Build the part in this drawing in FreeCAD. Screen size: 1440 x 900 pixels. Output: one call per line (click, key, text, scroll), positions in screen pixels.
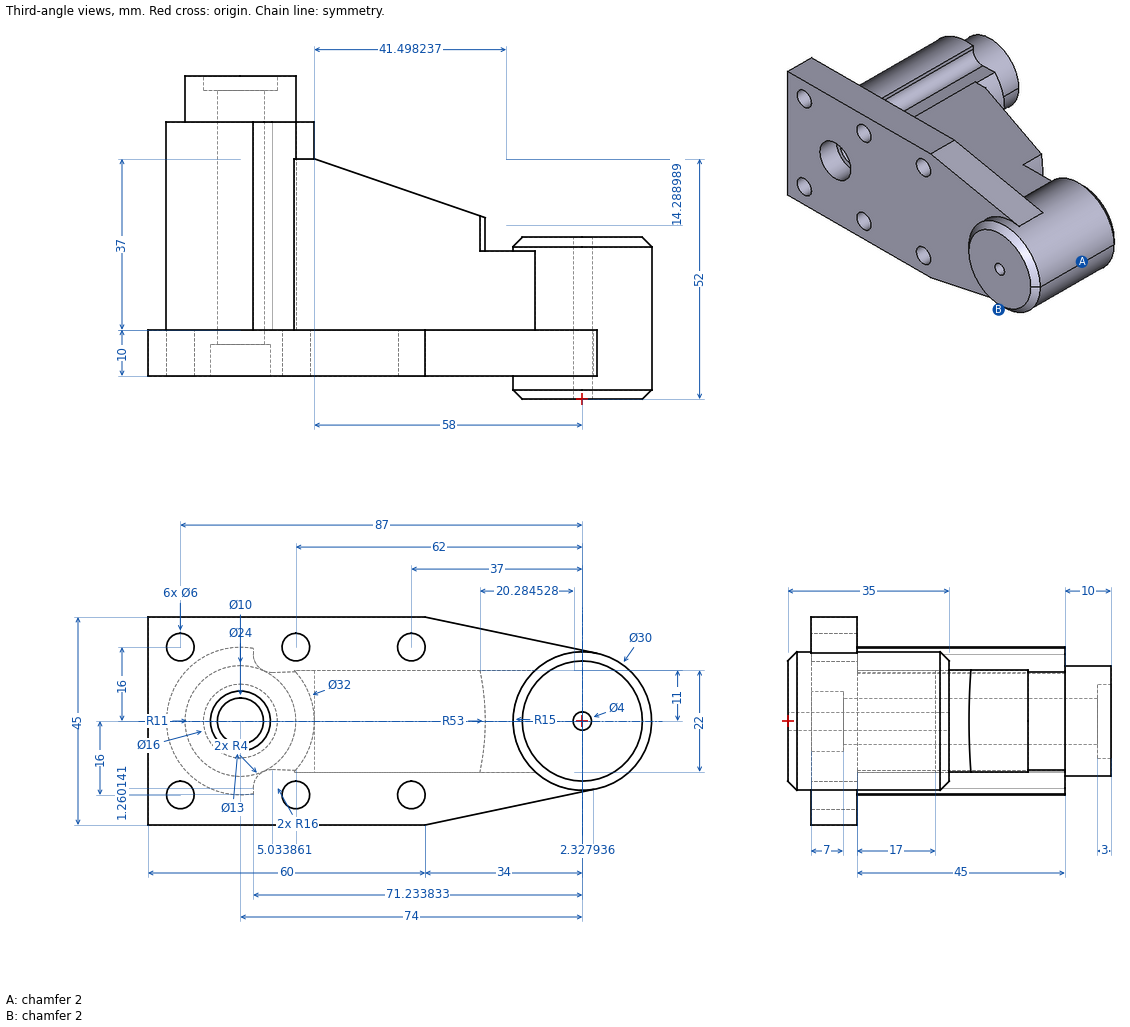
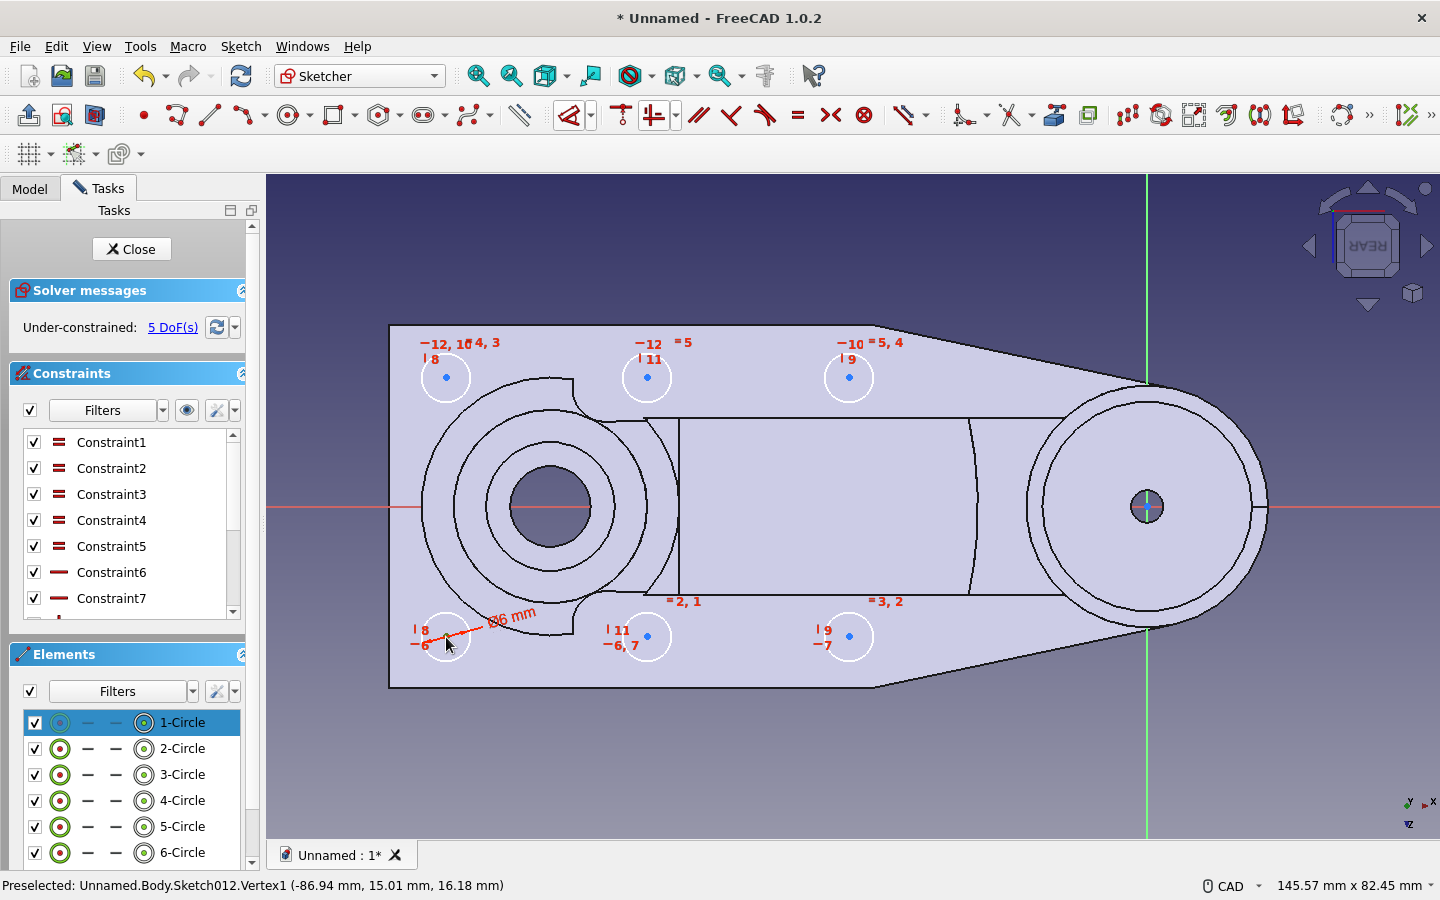
key(l)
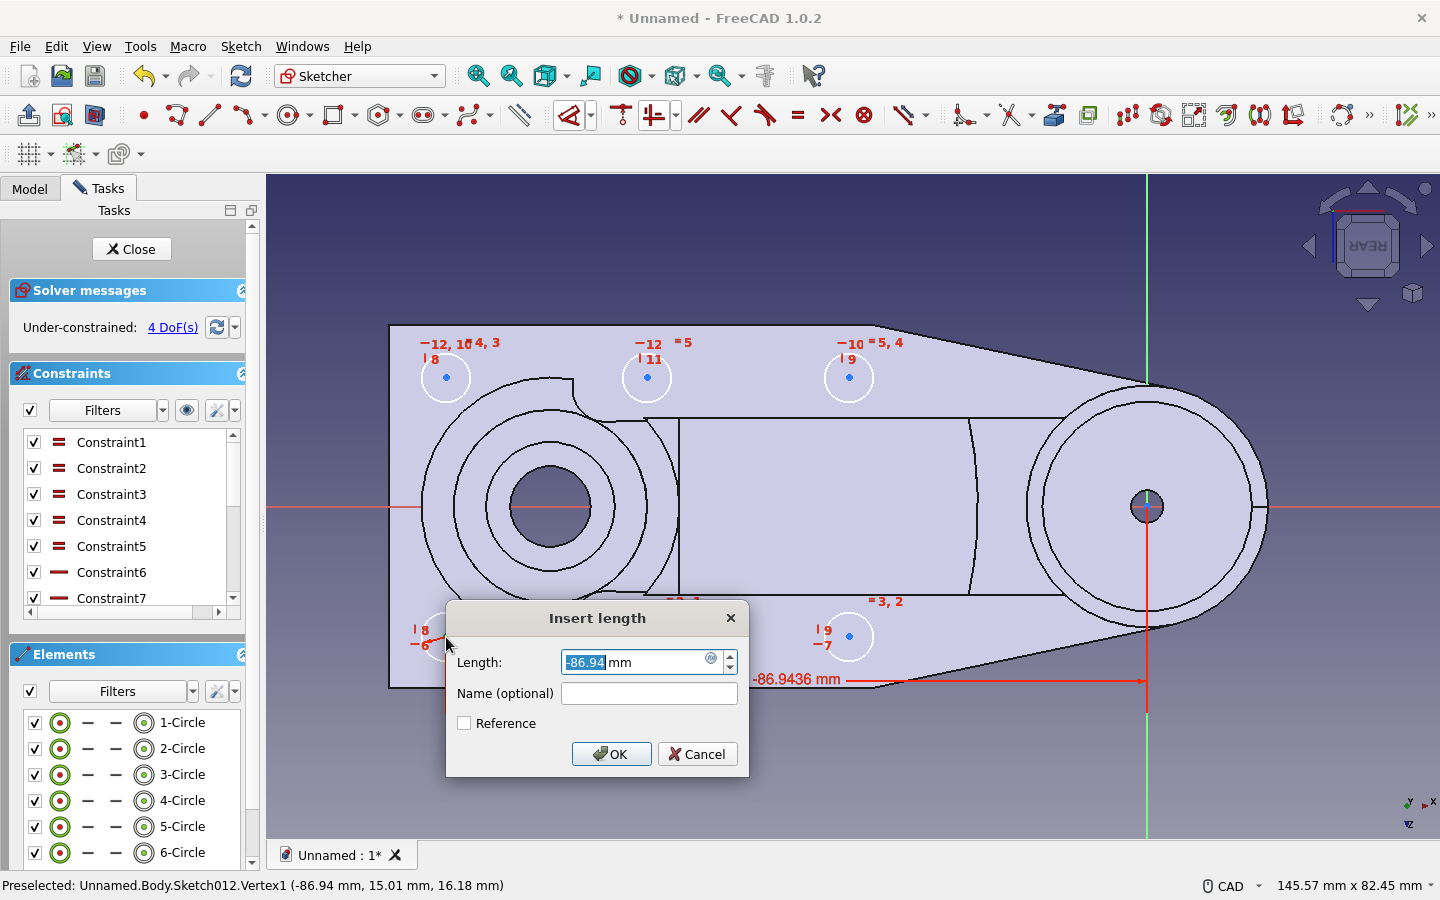
text(-87)
key(Return)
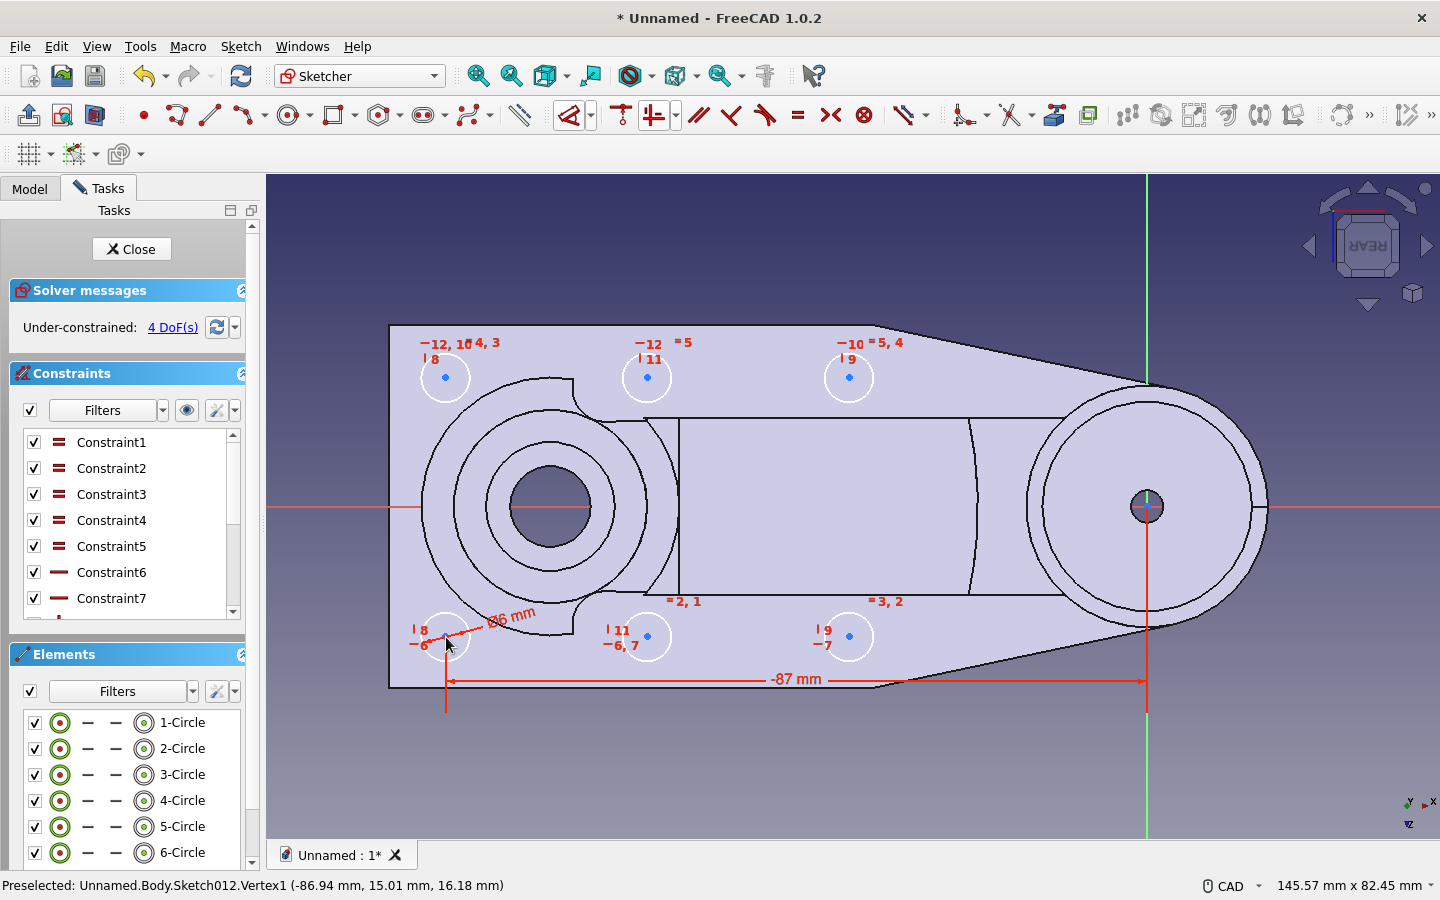
click(446, 637)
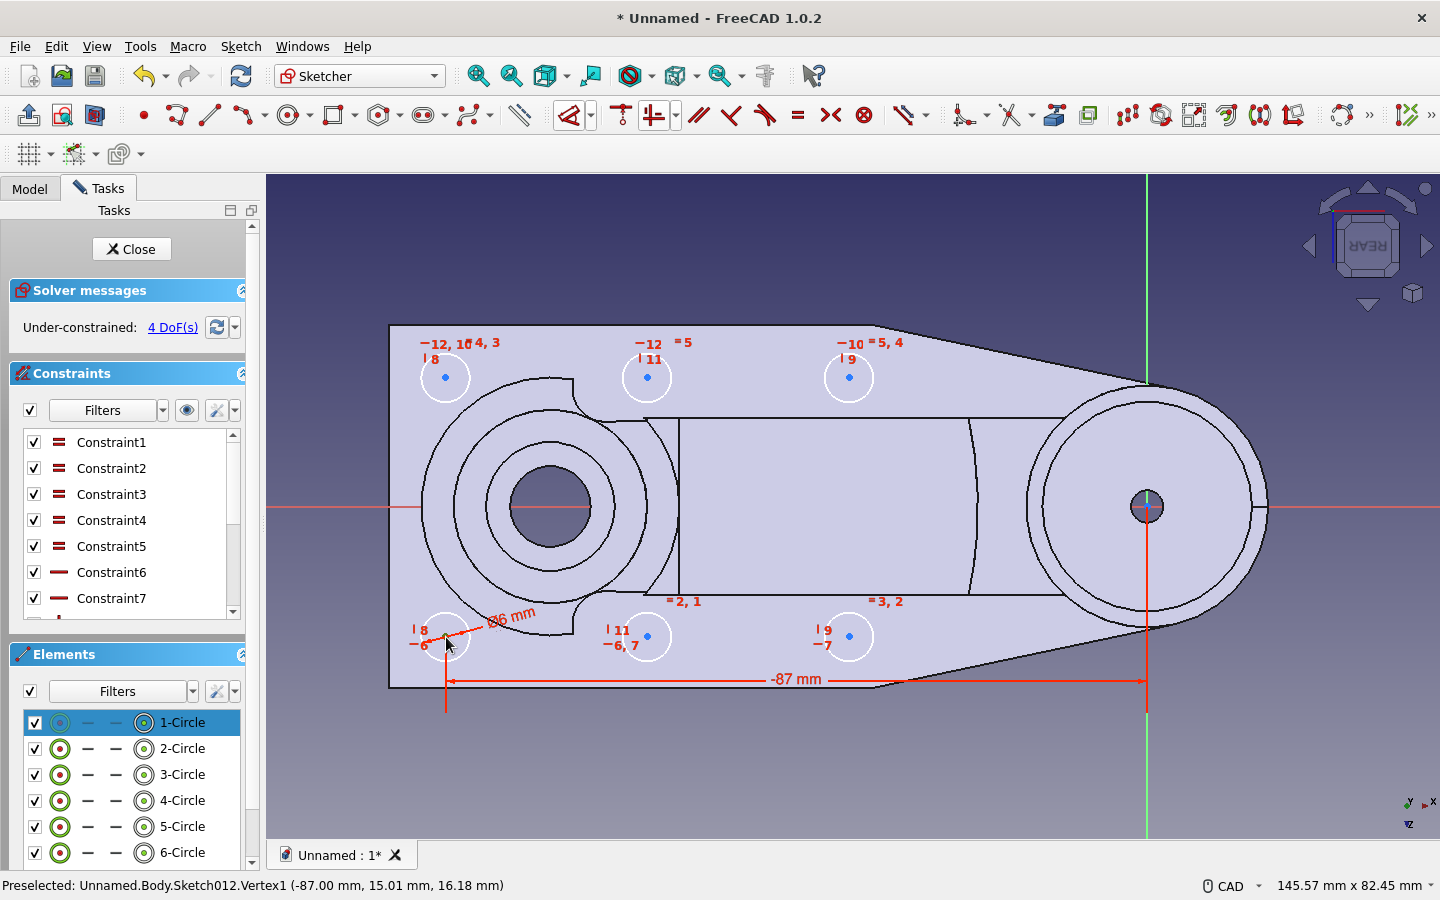
key(i)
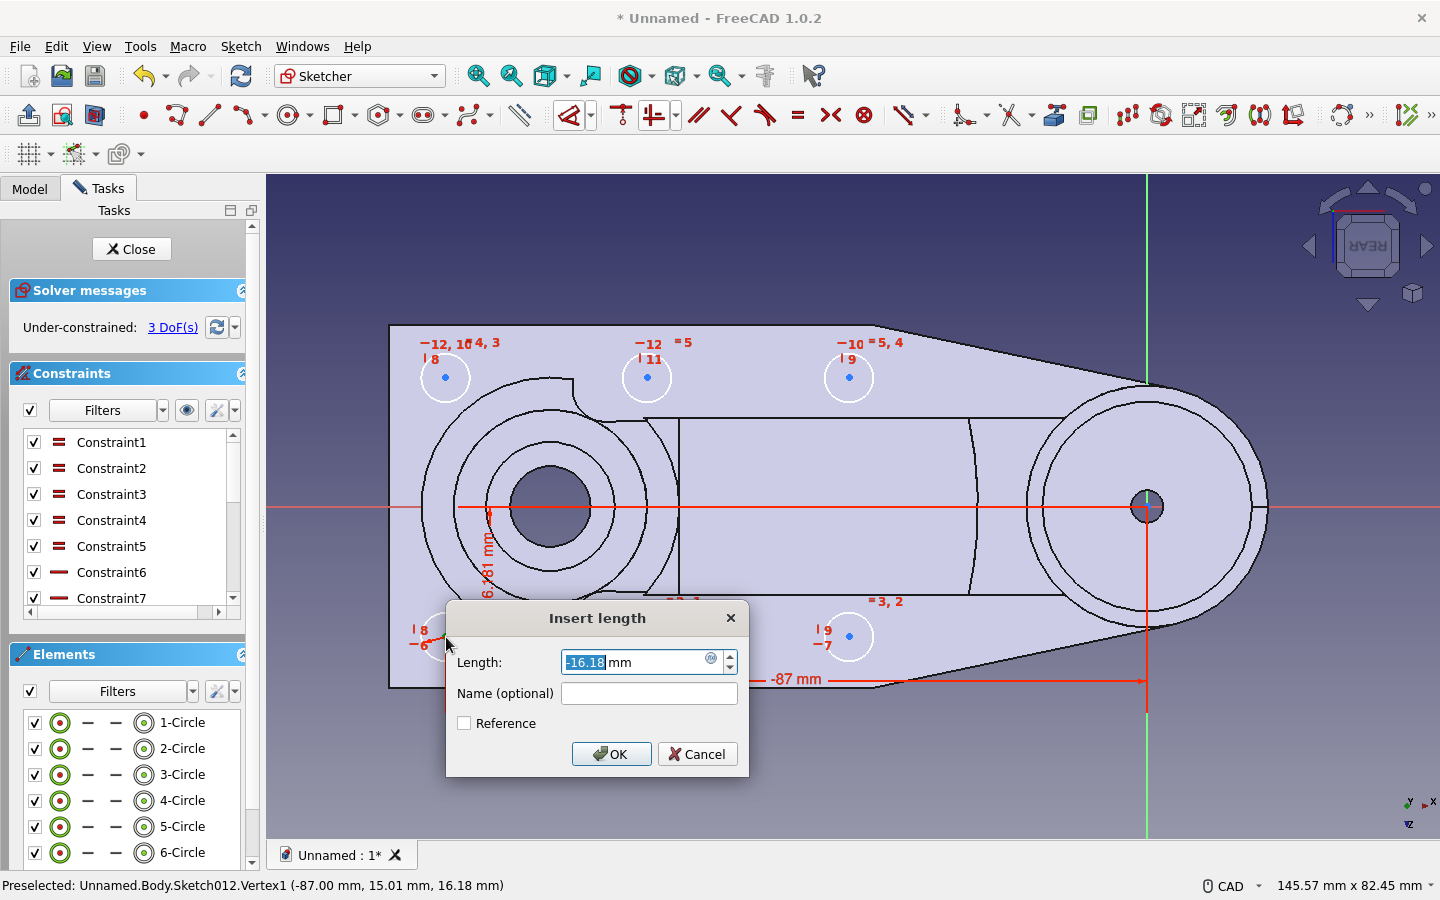
text(-16)
key(Return)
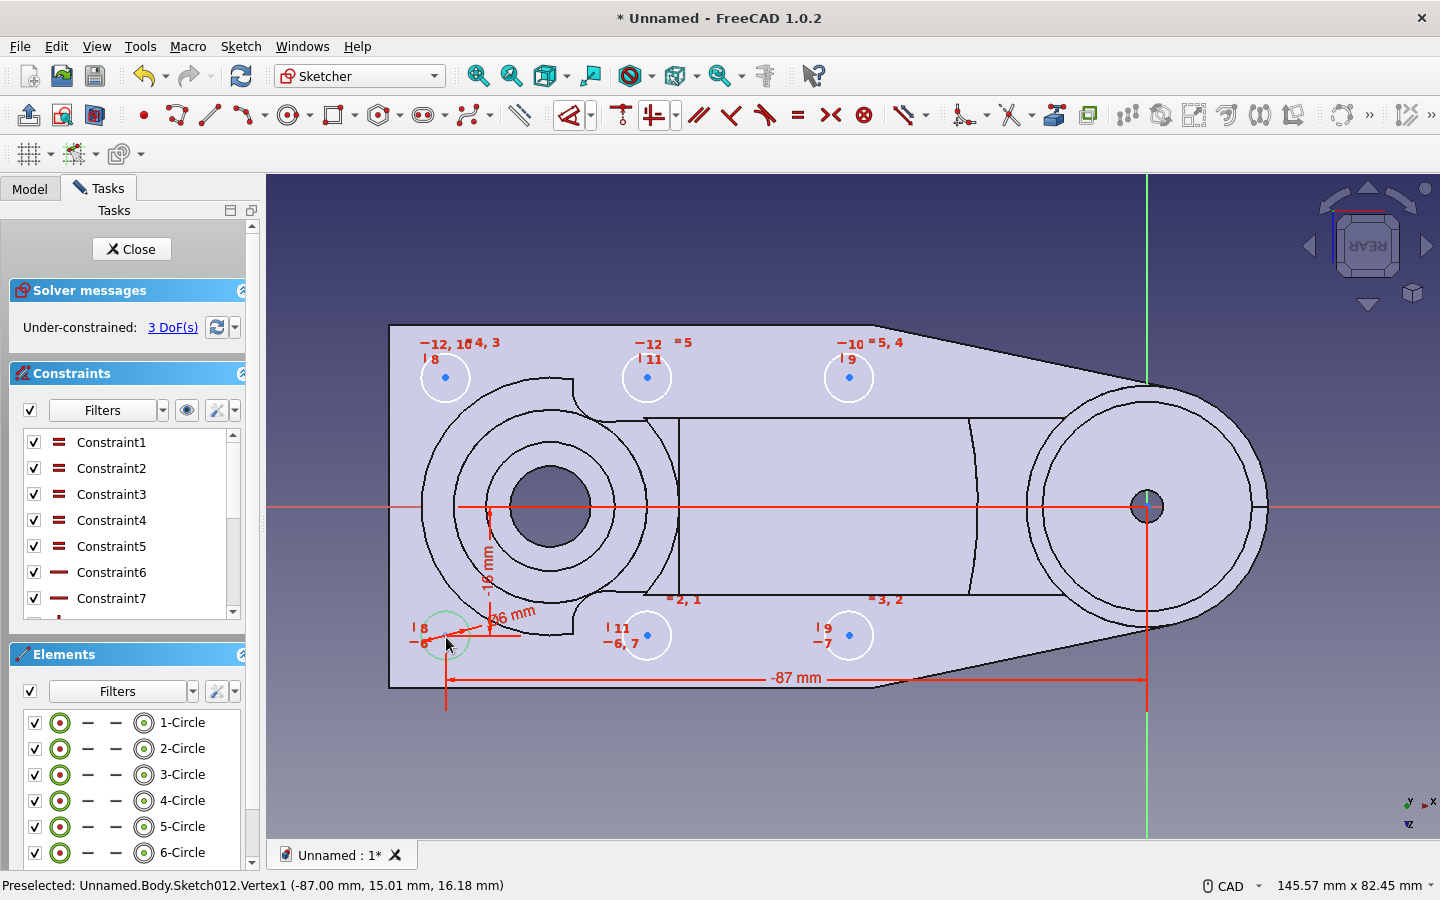
click(647, 636)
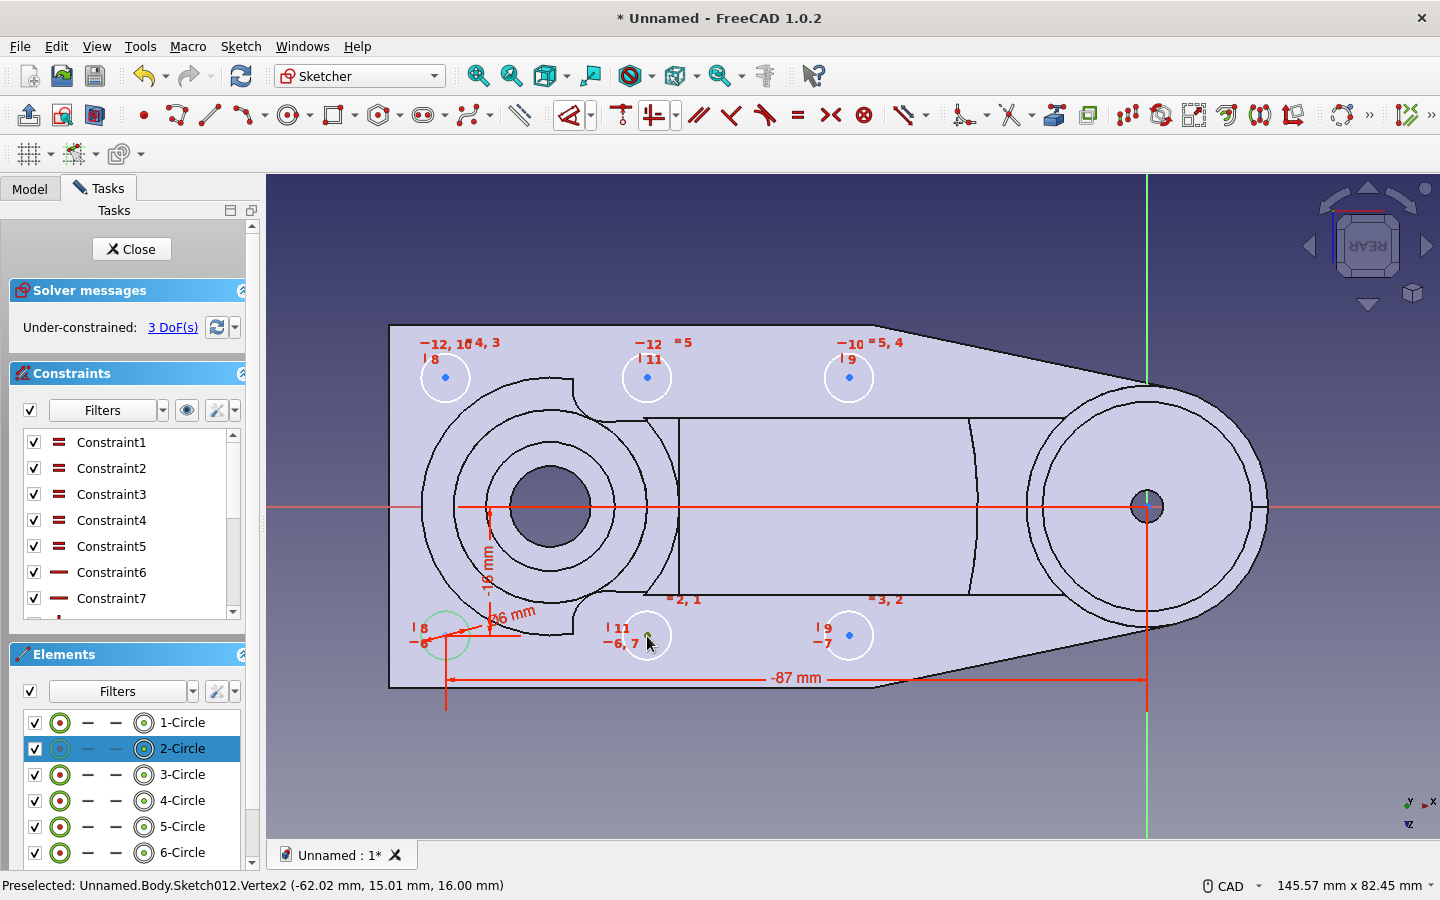
click(590, 116)